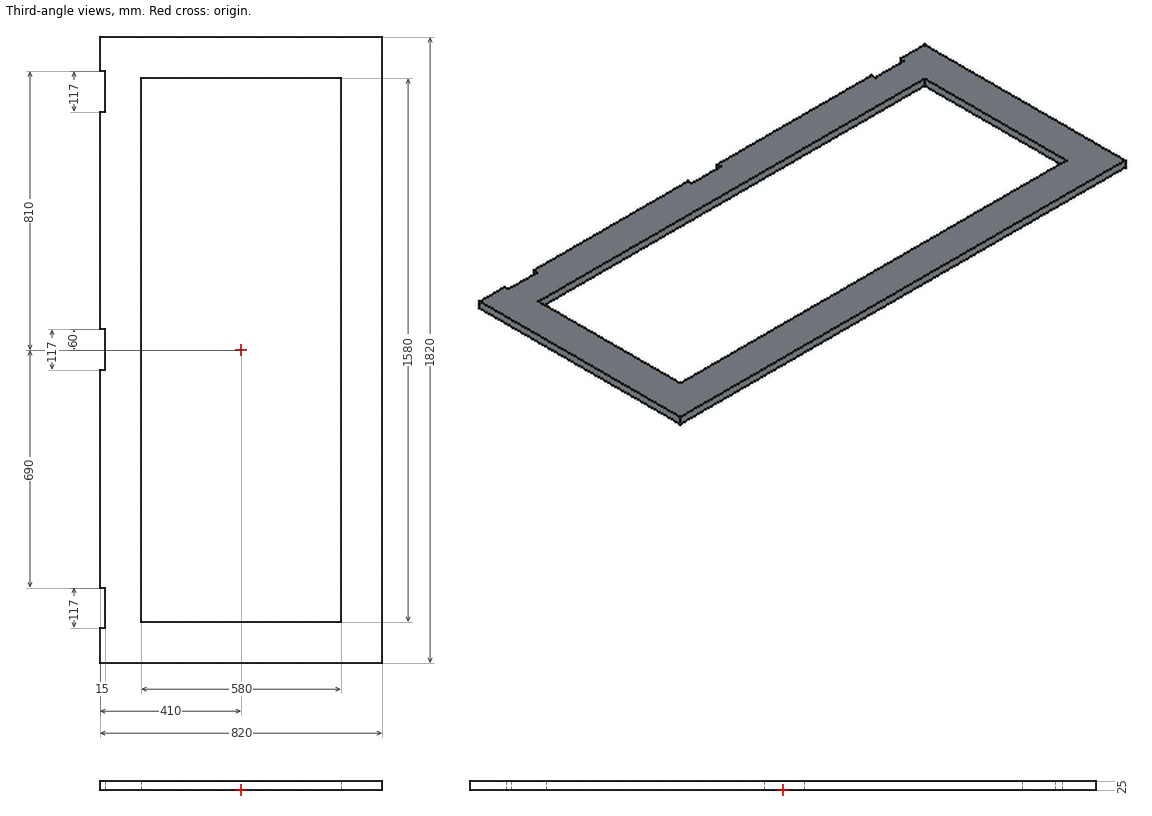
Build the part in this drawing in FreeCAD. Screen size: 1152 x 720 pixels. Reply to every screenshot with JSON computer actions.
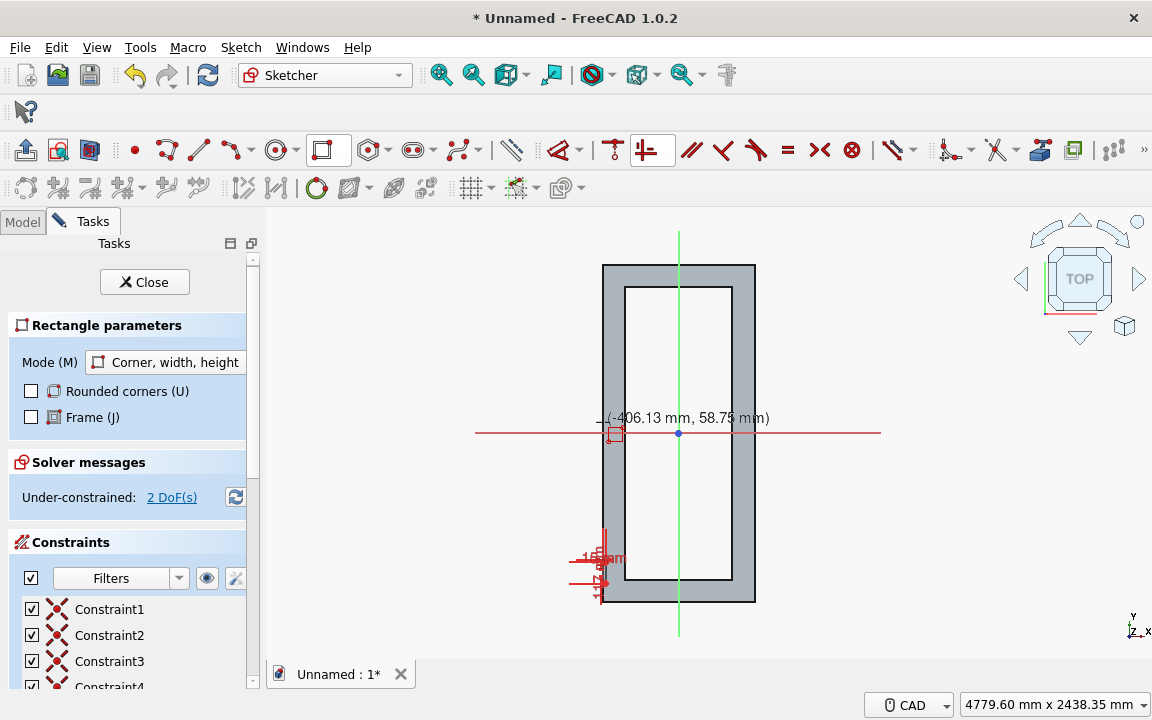
{"action": "scroll", "coordinate": [603, 422], "scroll_direction": "up", "scroll_amount": 2}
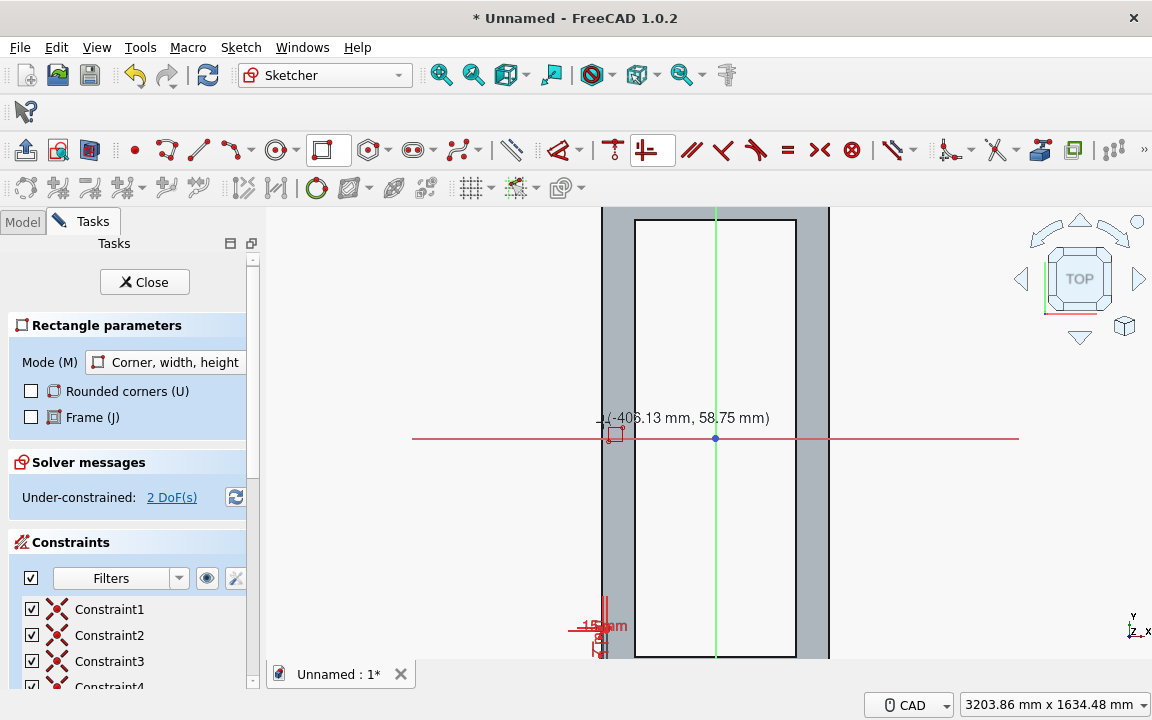
{"action": "left_click", "coordinate": [602, 422]}
{"action": "mouse_move", "coordinate": [606, 455]}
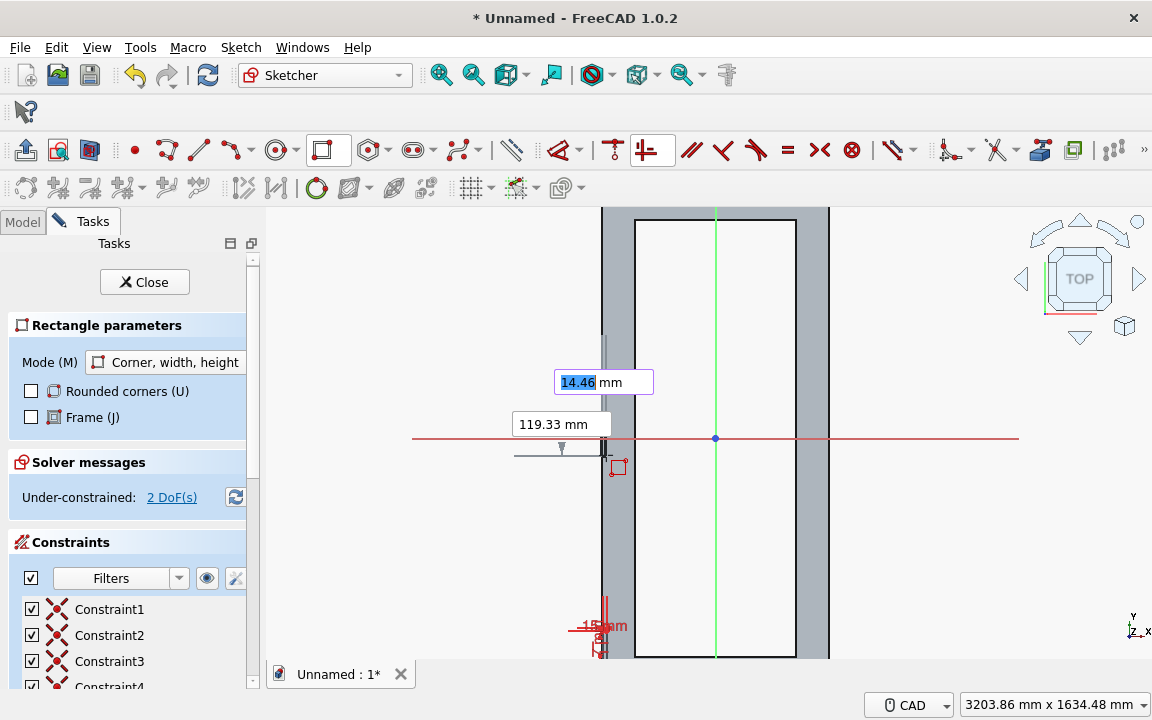
{"action": "type", "text": "15"}
{"action": "key", "text": "Tab"}
{"action": "type", "text": "117"}
{"action": "key", "text": "Return"}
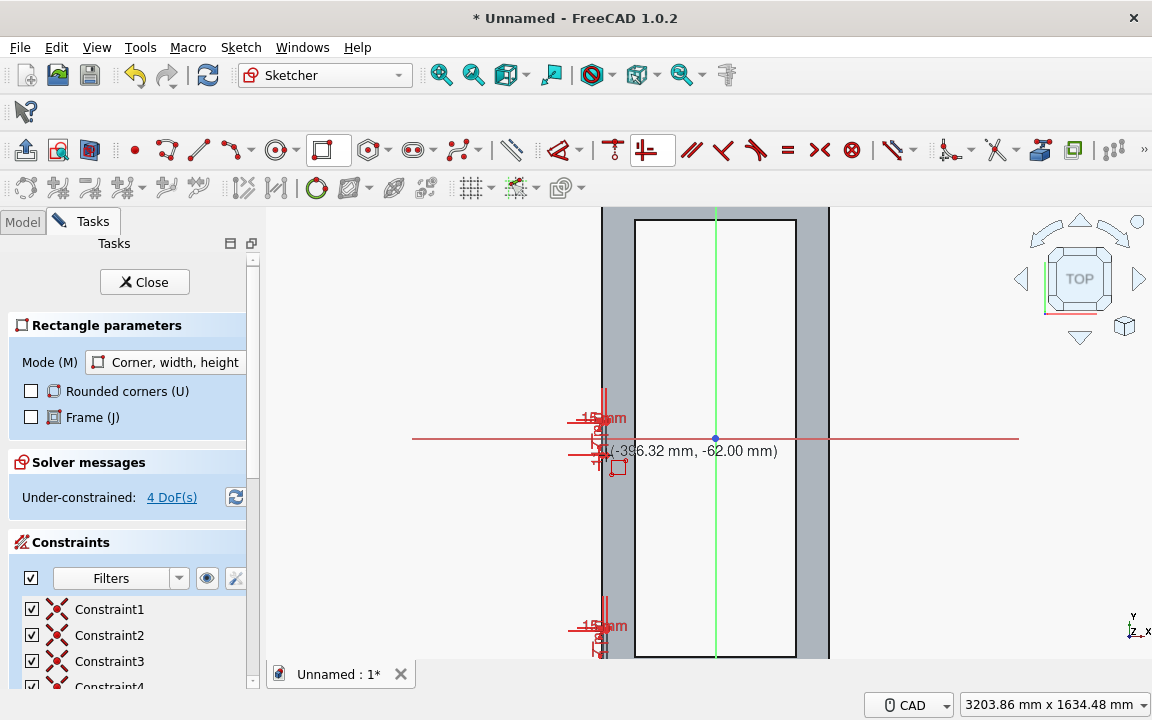
{"action": "scroll", "coordinate": [603, 422], "scroll_direction": "down", "scroll_amount": 2}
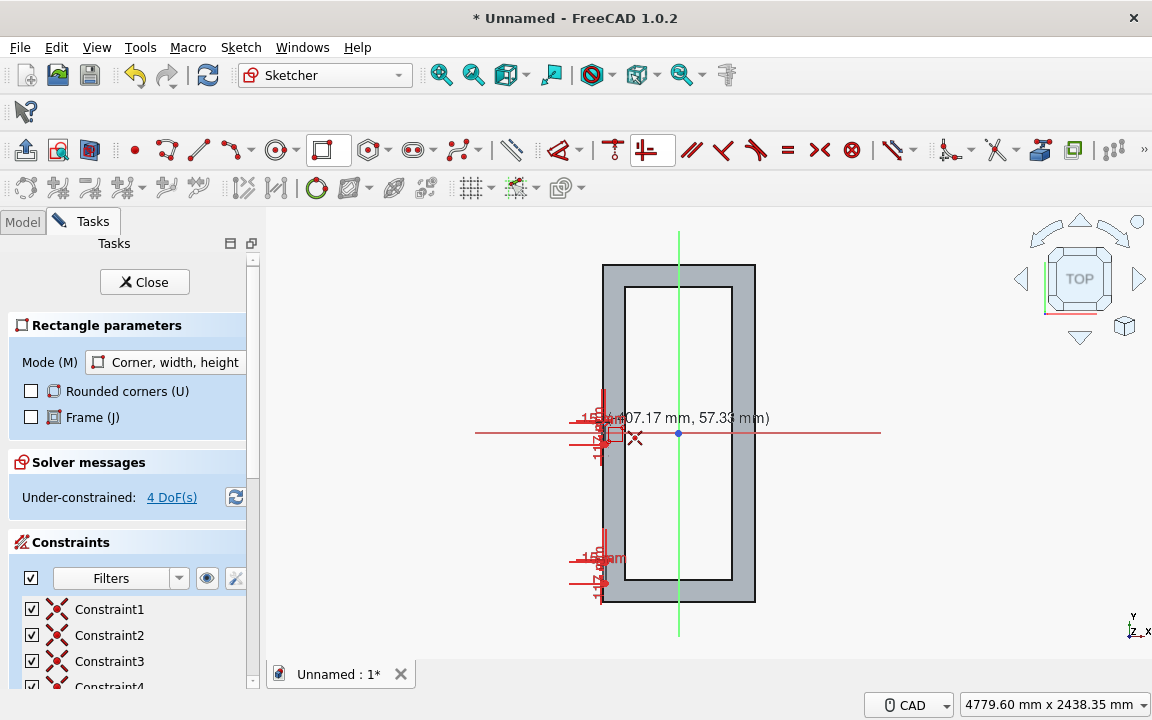
{"action": "scroll", "coordinate": [603, 283], "scroll_direction": "up", "scroll_amount": 9}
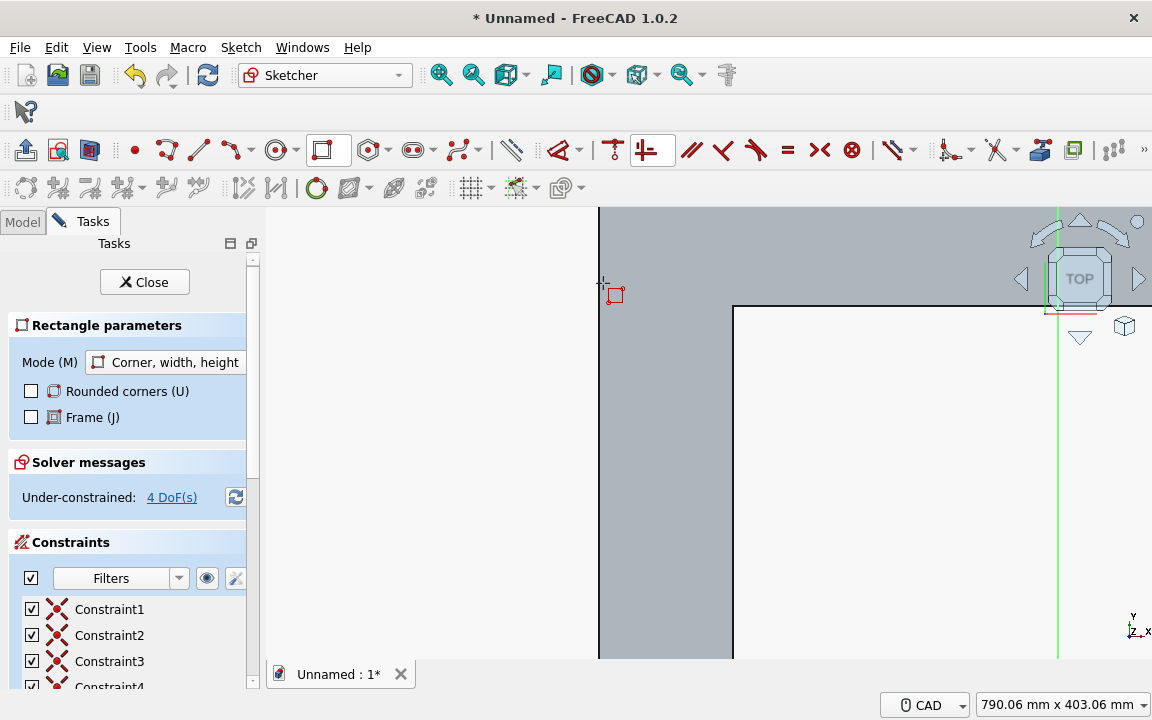
{"action": "scroll", "coordinate": [603, 283], "scroll_direction": "down", "scroll_amount": 9}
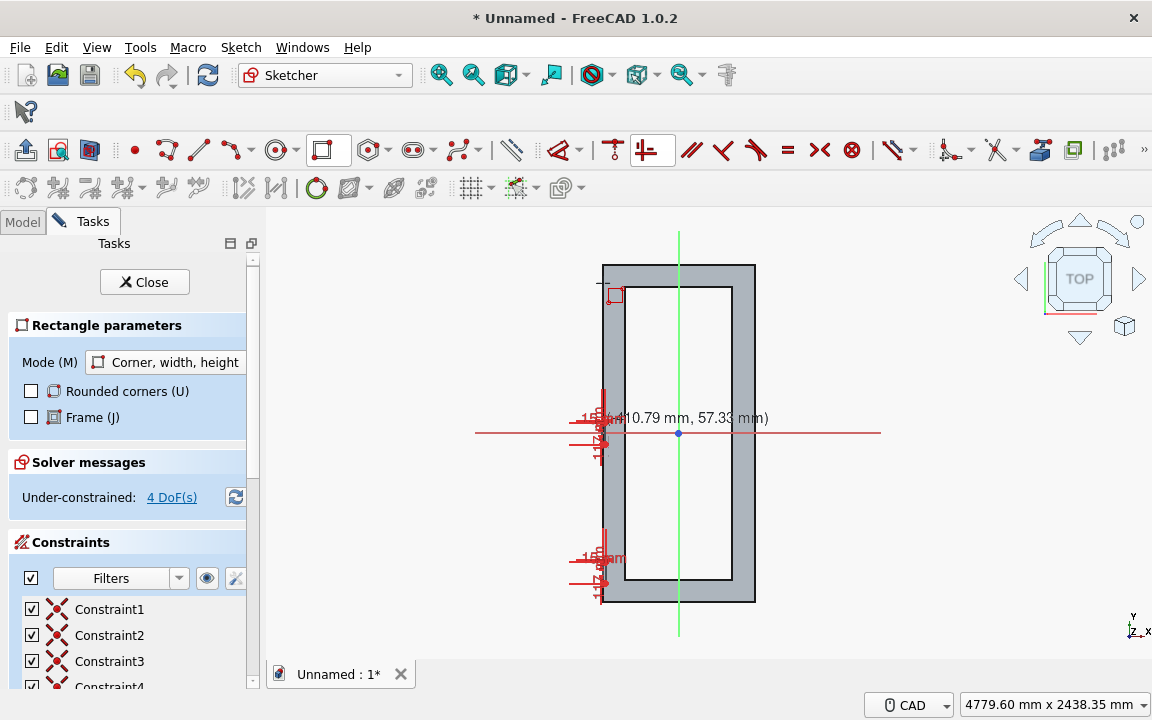
{"action": "left_click", "coordinate": [603, 283]}
{"action": "mouse_move", "coordinate": [605, 305]}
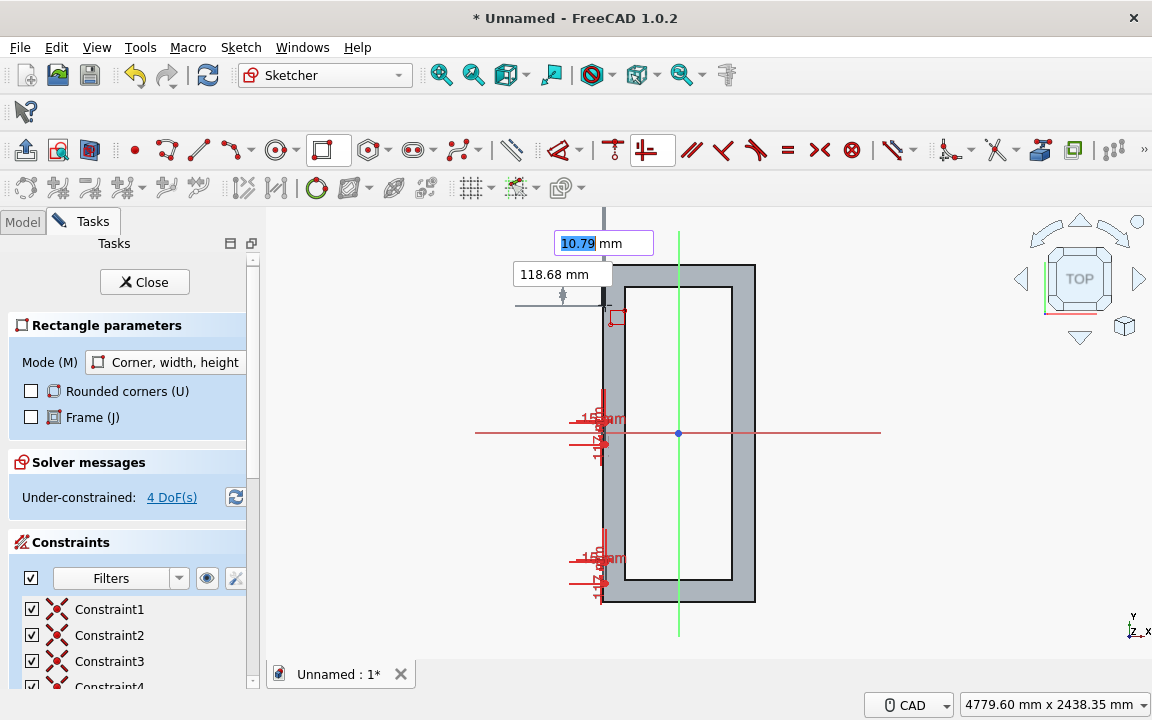
{"action": "type", "text": "15"}
{"action": "key", "text": "Tab"}
{"action": "type", "text": "117"}
{"action": "key", "text": "Return"}
{"action": "key", "text": "Escape"}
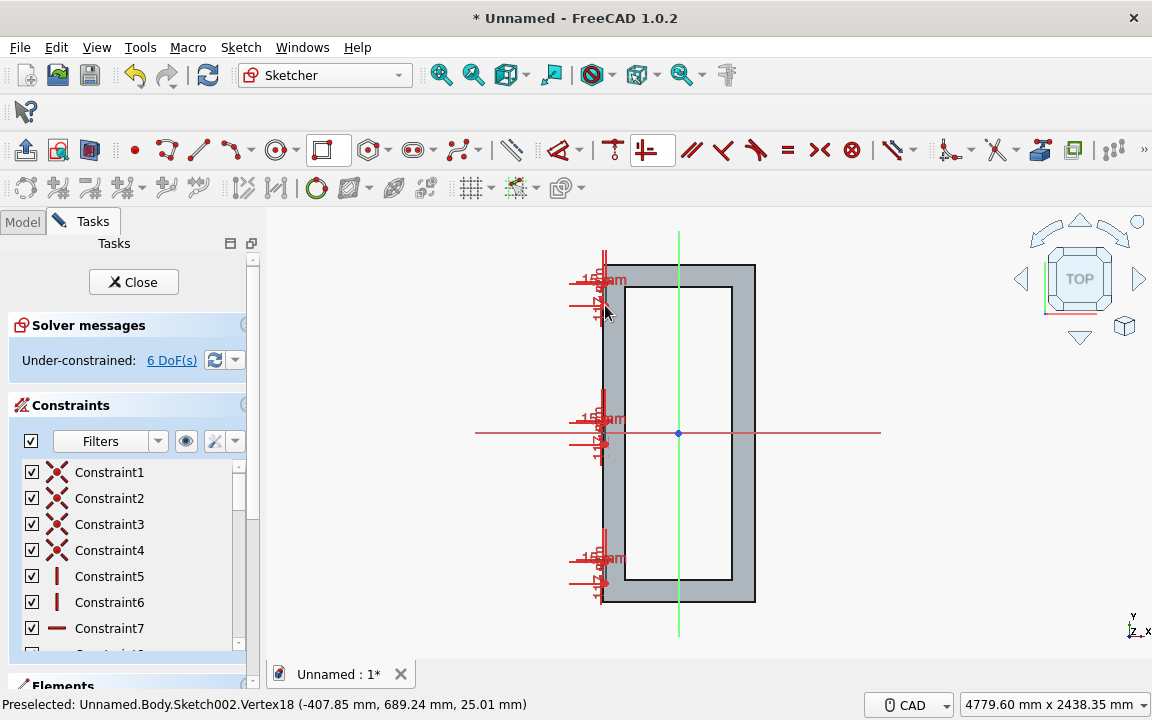
{"action": "left_click", "coordinate": [558, 150]}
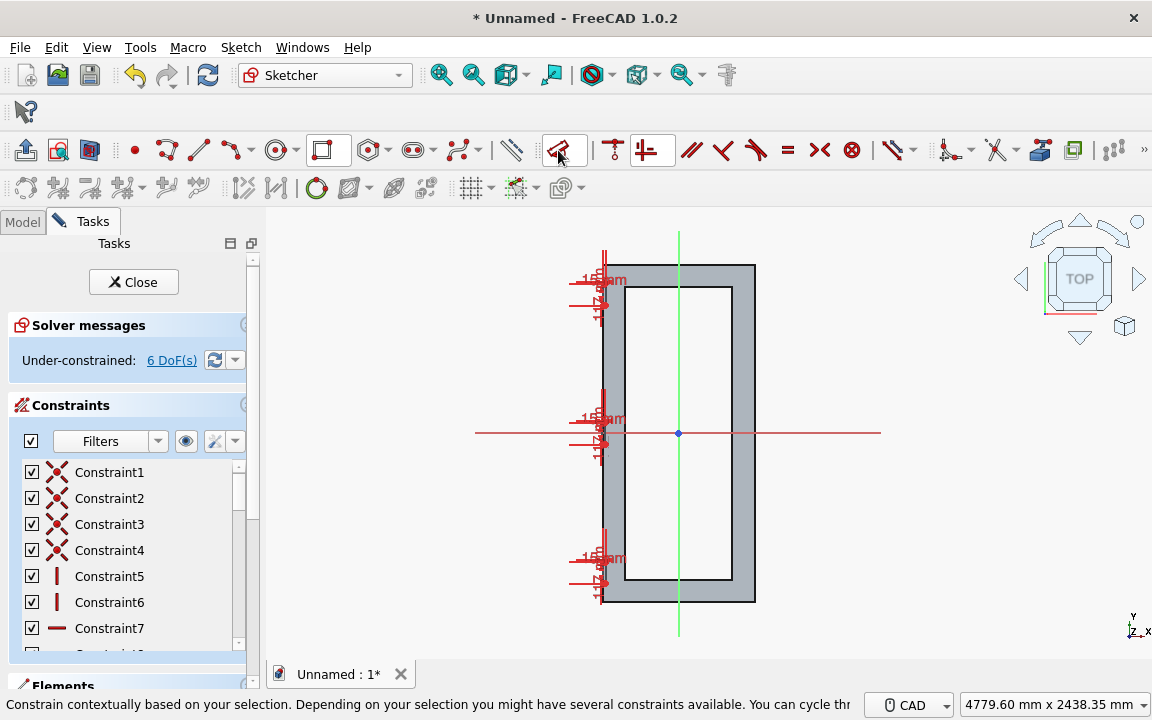
{"action": "scroll", "coordinate": [602, 423], "scroll_direction": "up", "scroll_amount": 8}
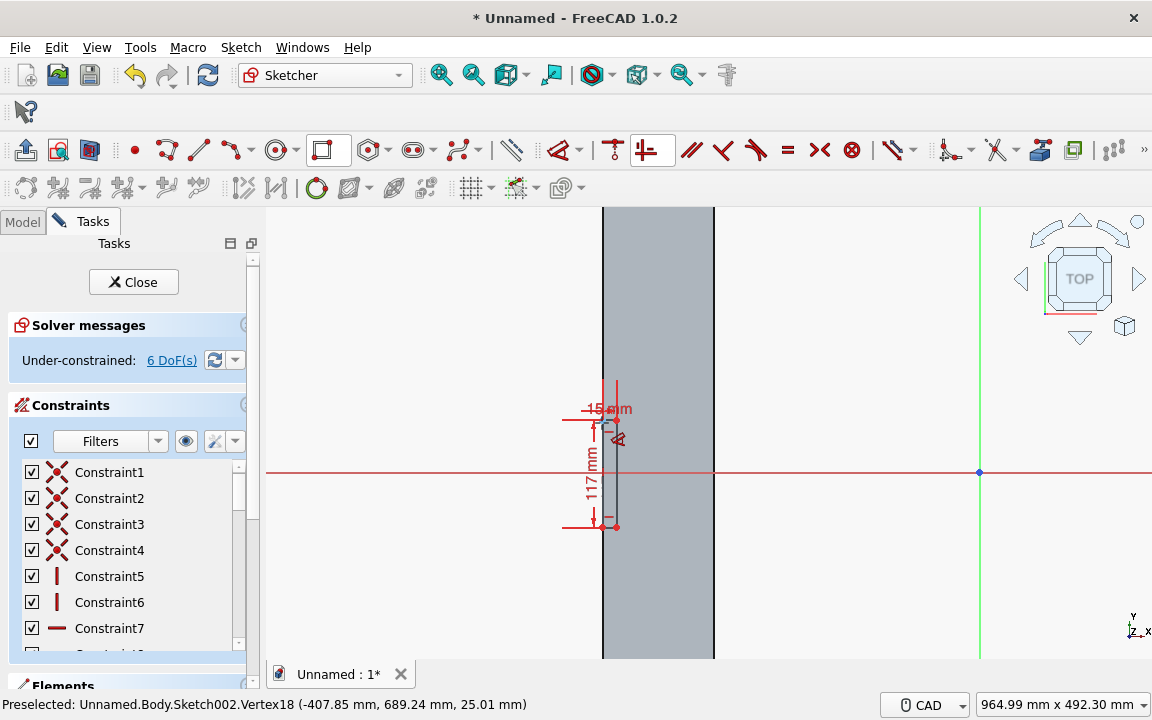
{"action": "left_click", "coordinate": [603, 420]}
{"action": "left_click", "coordinate": [569, 447]}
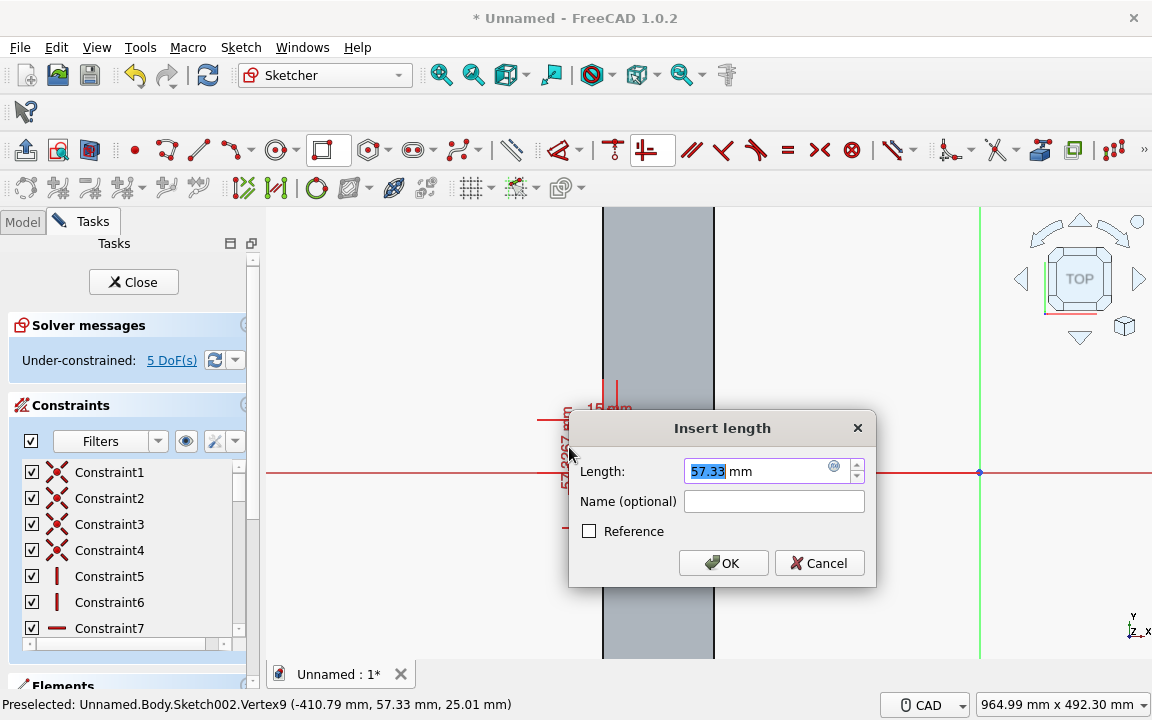
{"action": "type", "text": "60"}
{"action": "key", "text": "Return"}